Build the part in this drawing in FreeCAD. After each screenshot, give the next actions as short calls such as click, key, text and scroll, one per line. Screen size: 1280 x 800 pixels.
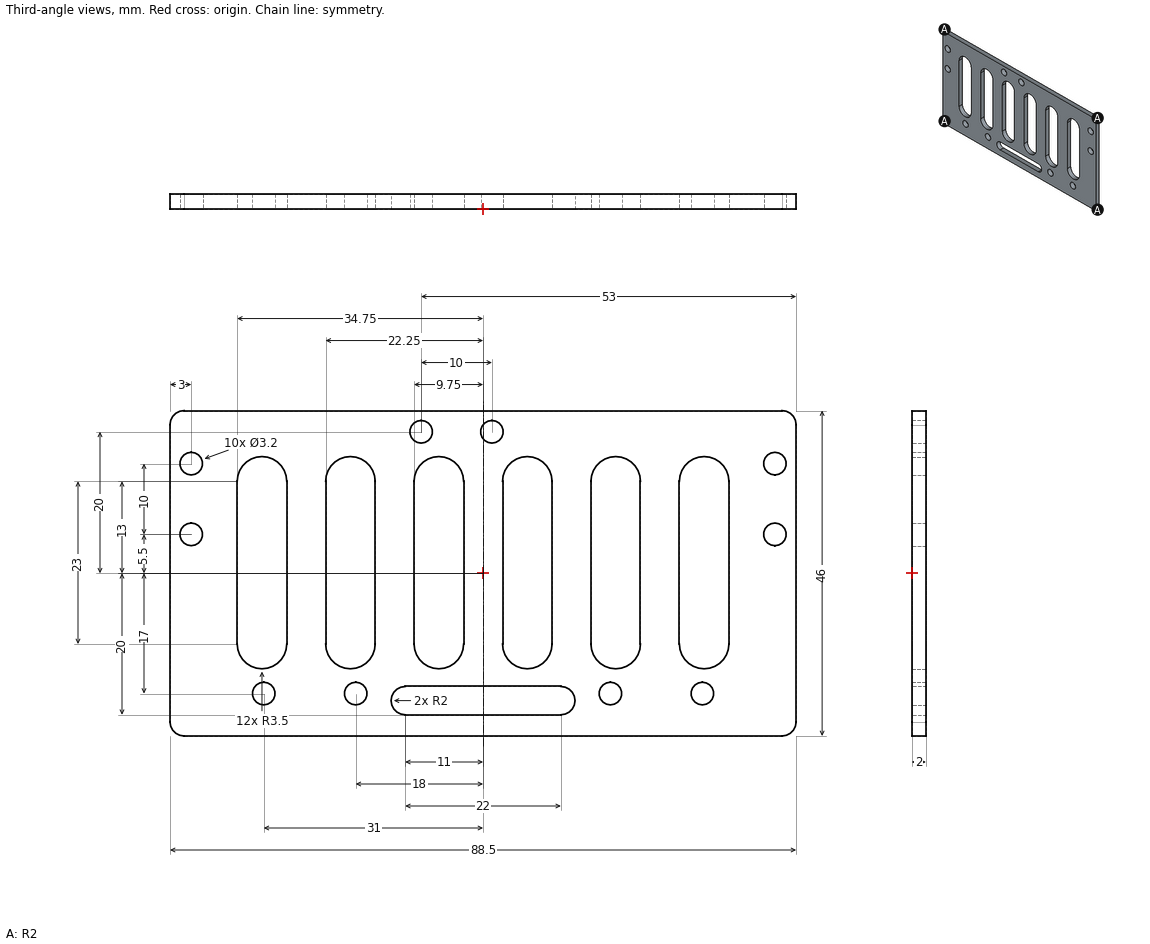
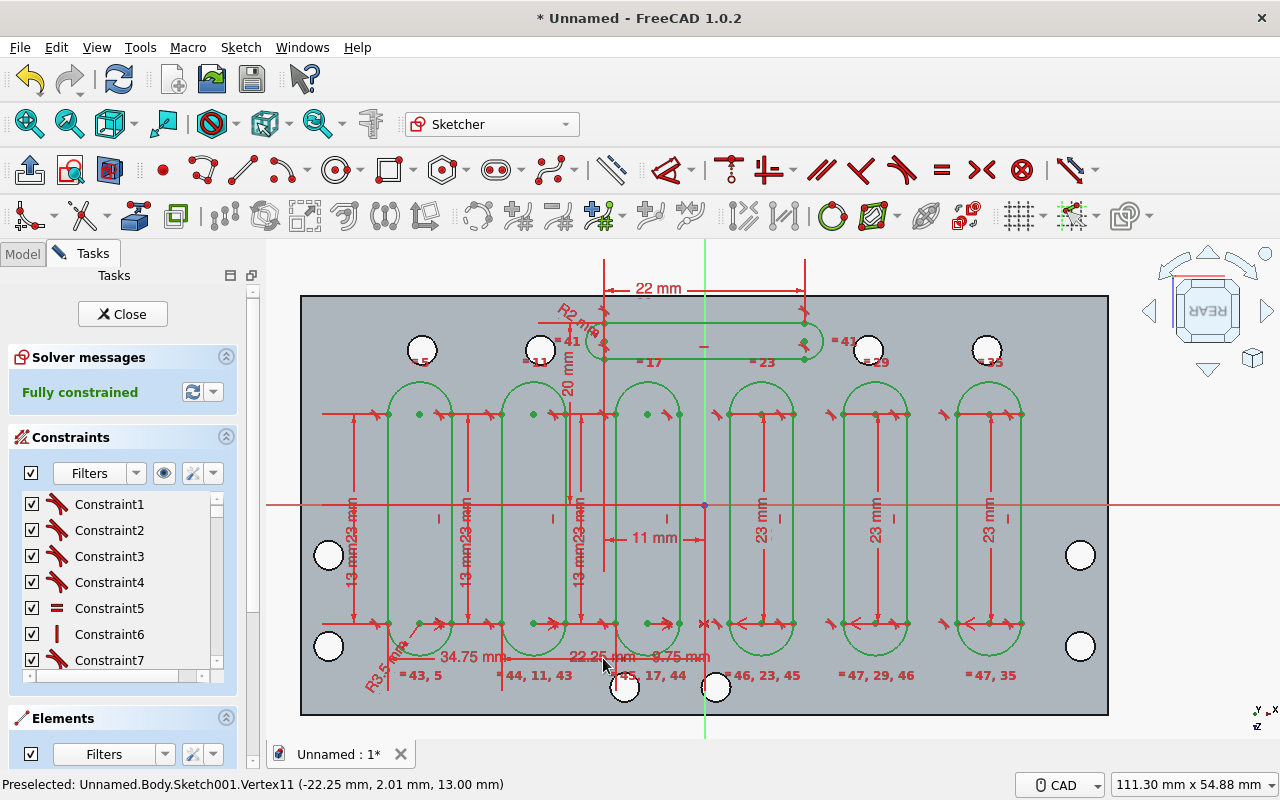
click(123, 314)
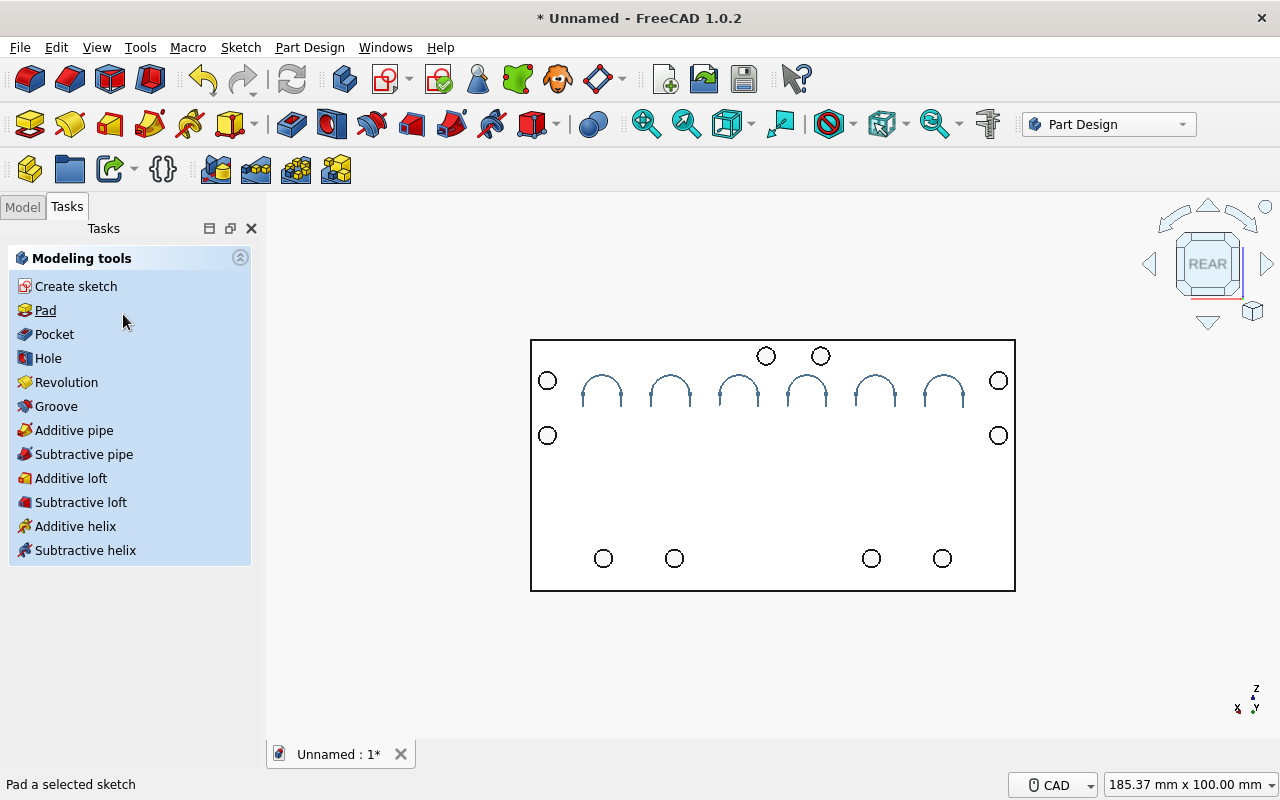
click(292, 124)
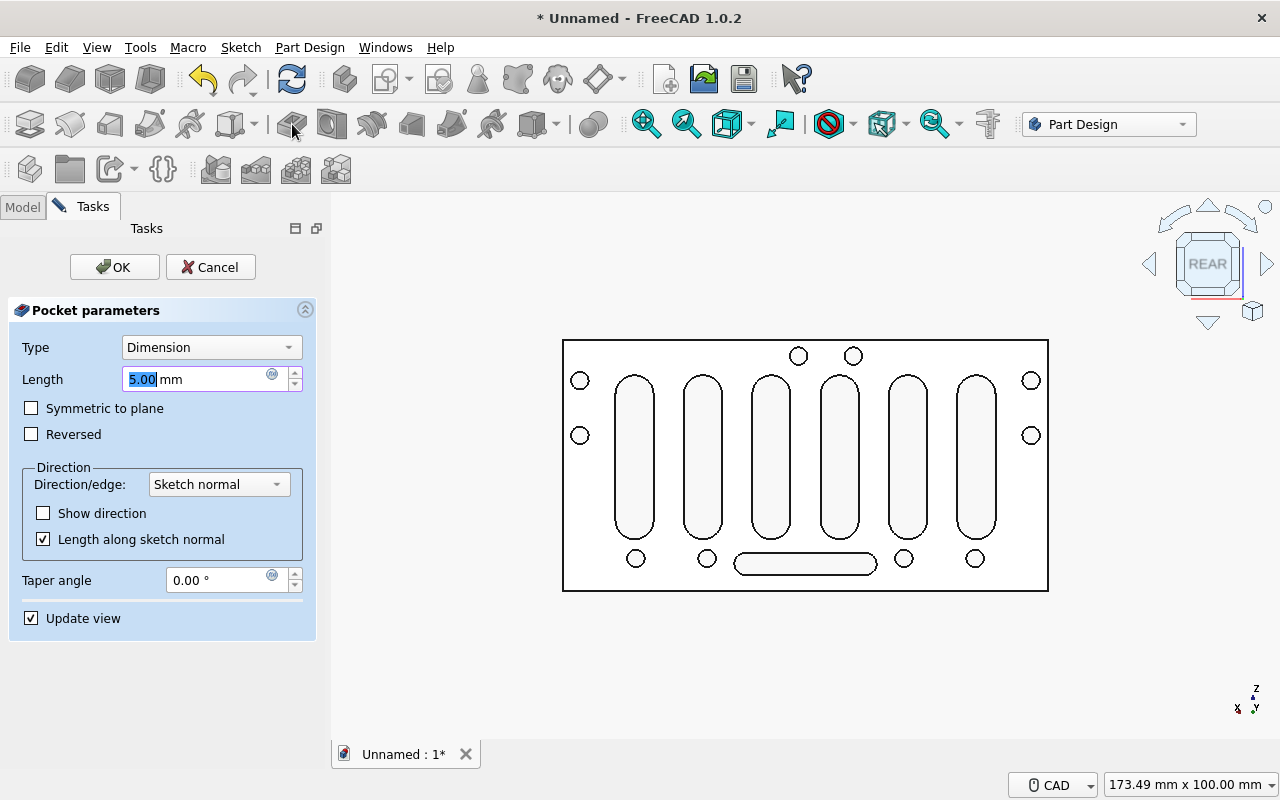
click(212, 348)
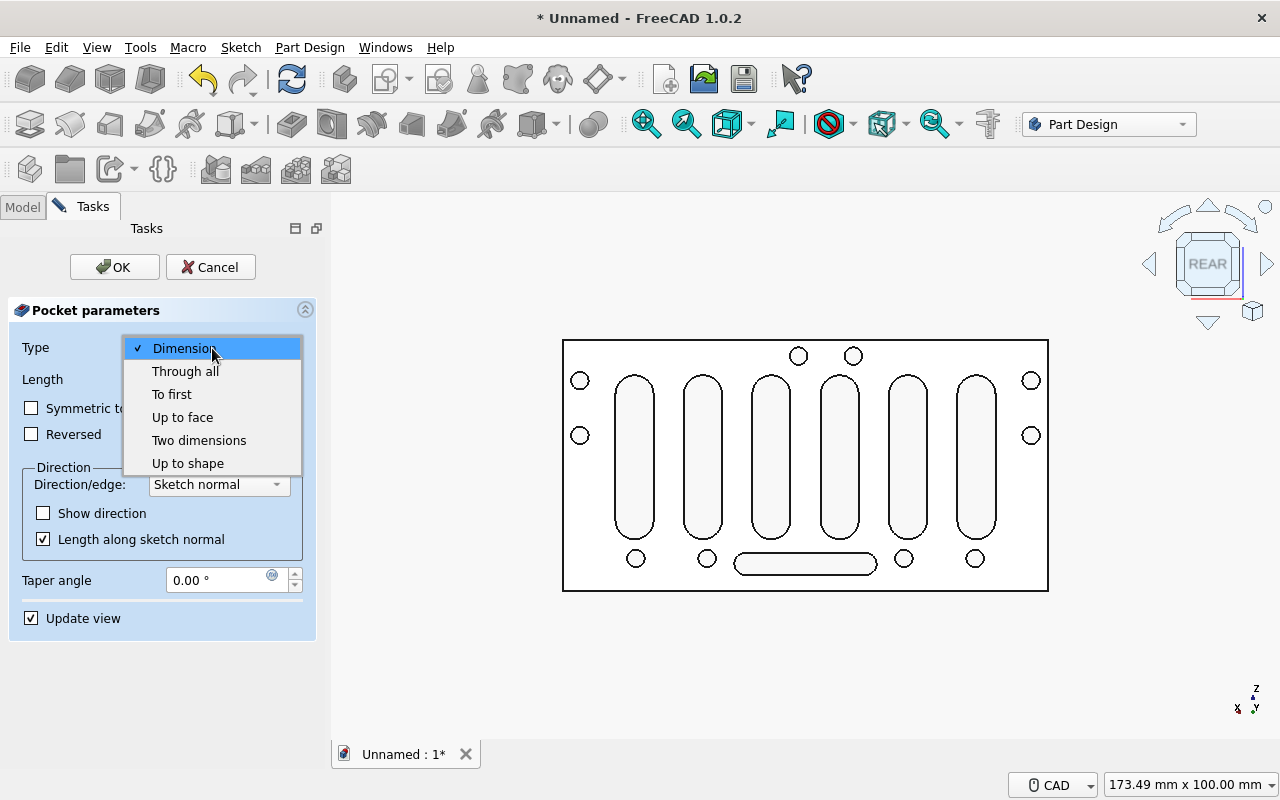
click(212, 372)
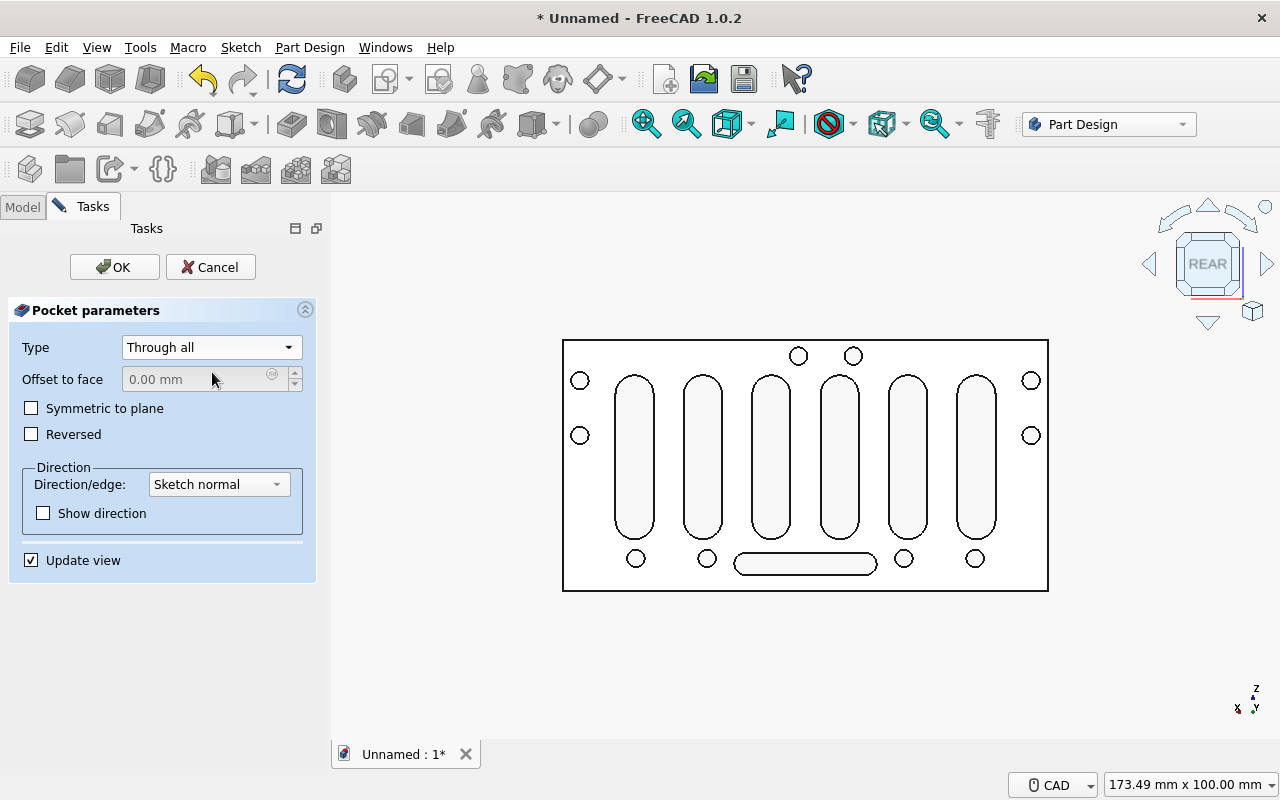
click(115, 267)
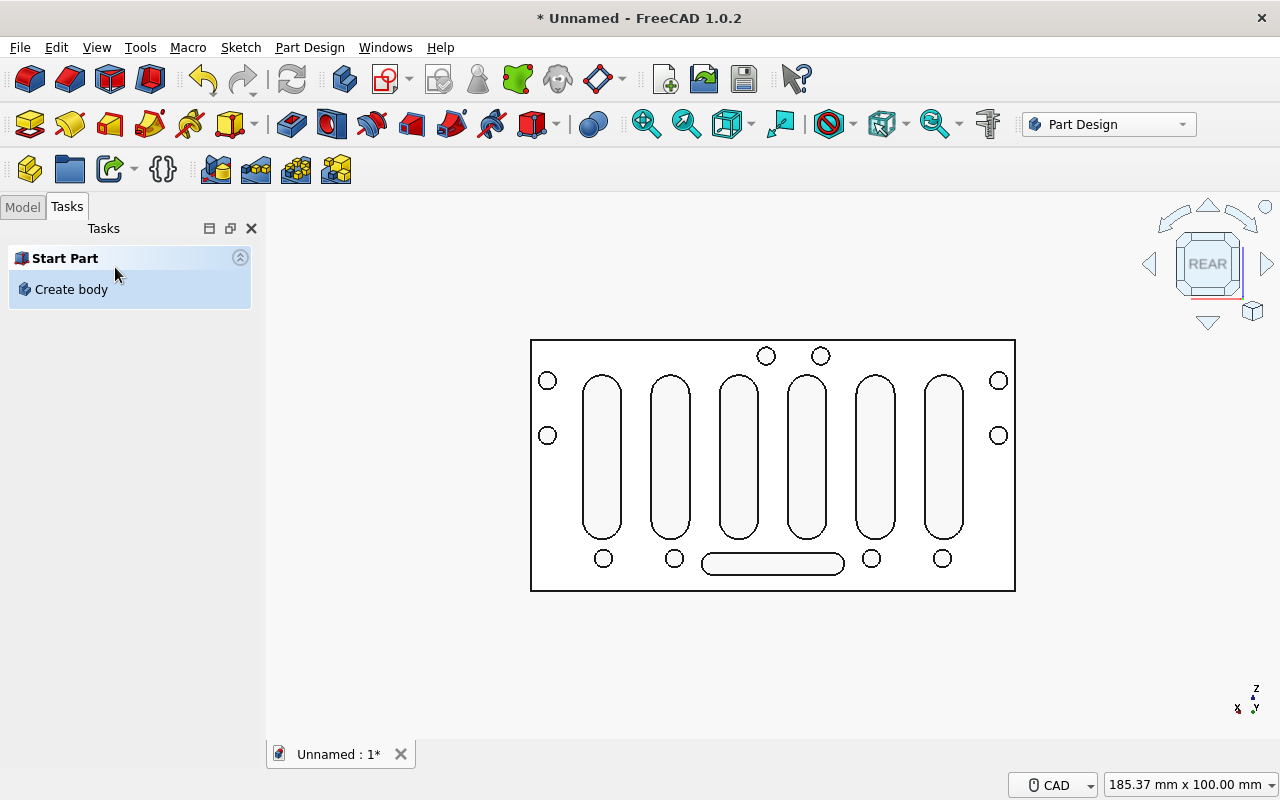
scroll(531, 339, up, 7)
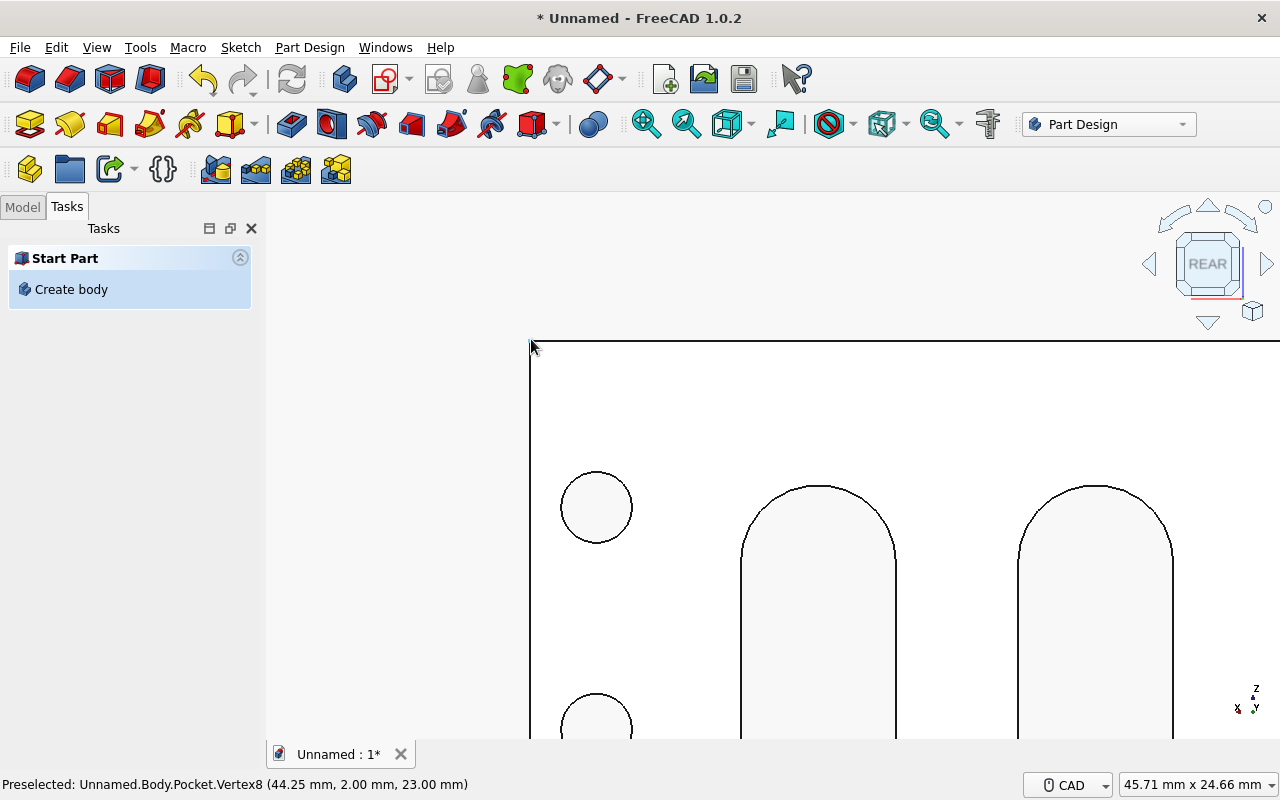
click(648, 124)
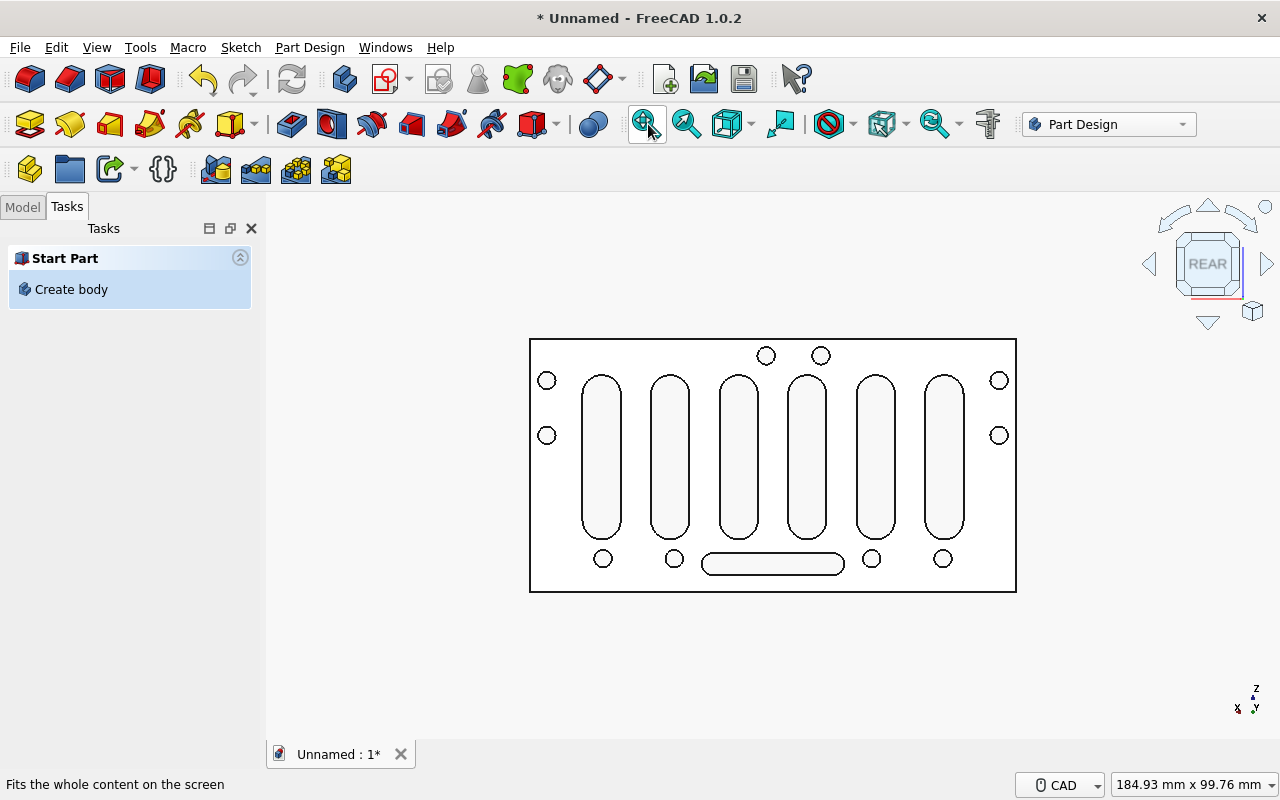
key(0)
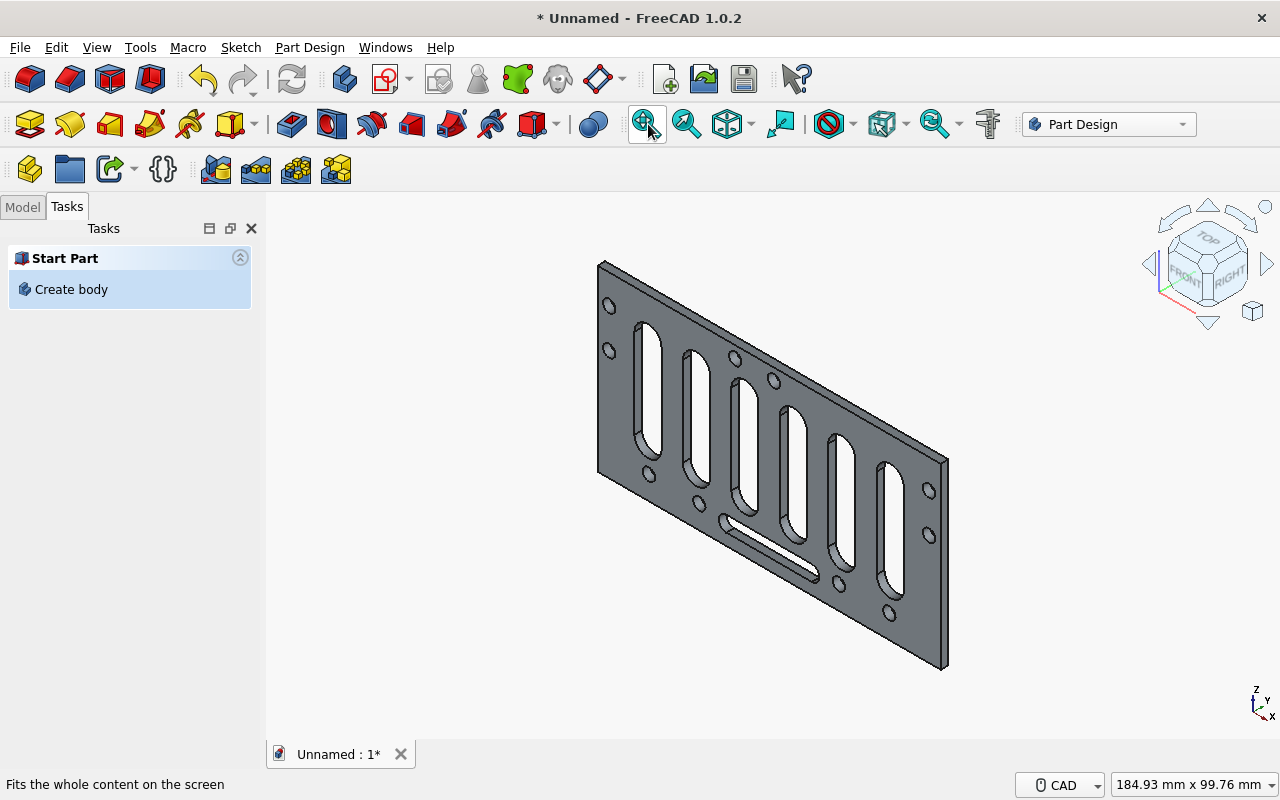
scroll(945, 461, up, 7)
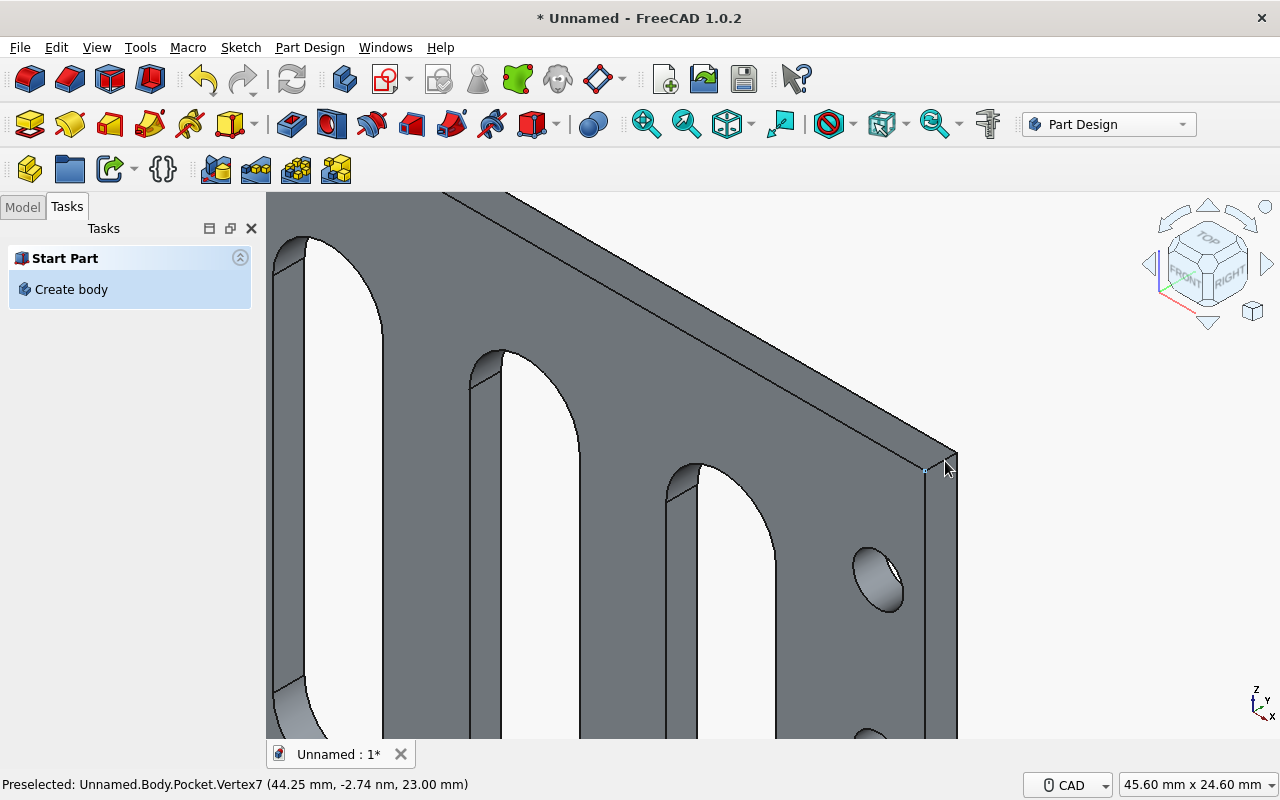
click(941, 461)